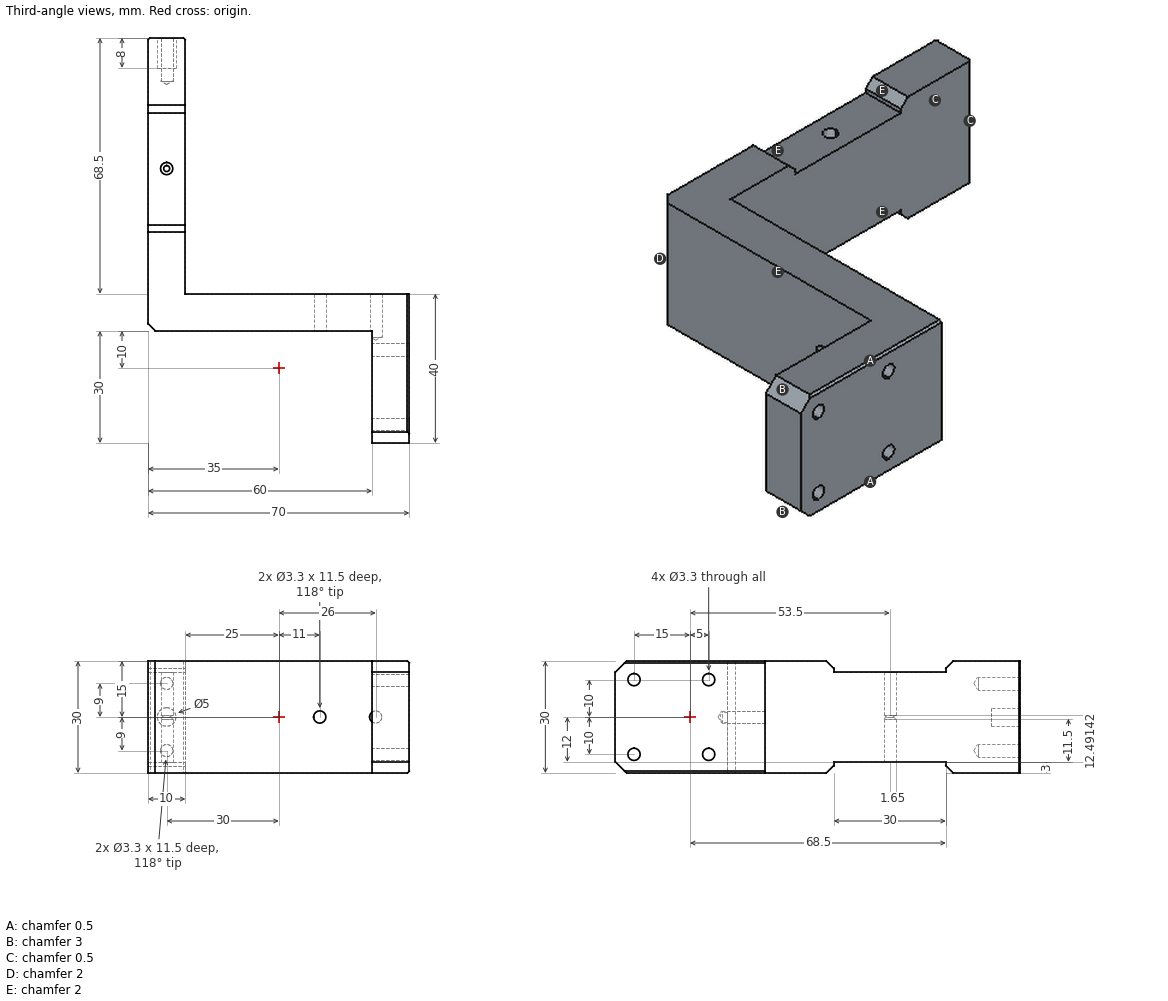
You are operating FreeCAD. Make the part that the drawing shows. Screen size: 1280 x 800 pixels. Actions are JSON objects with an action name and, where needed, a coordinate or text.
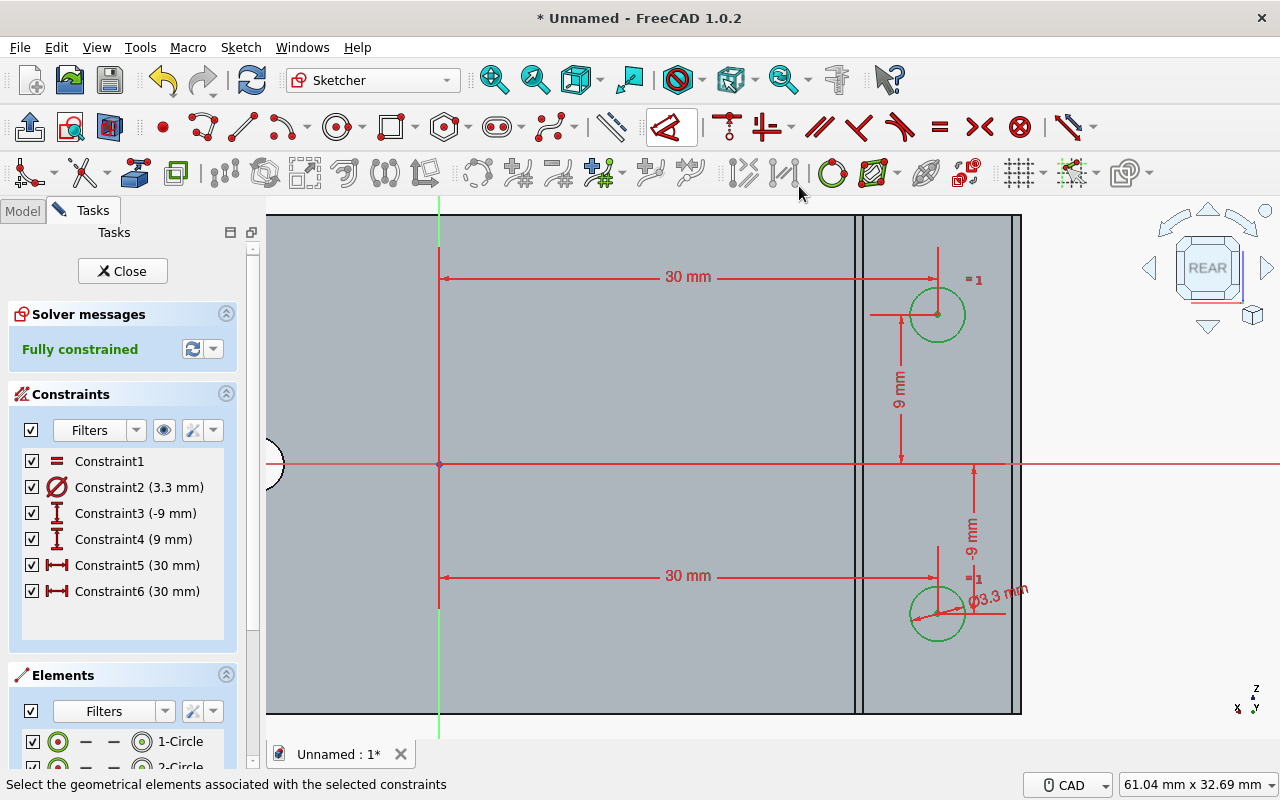
{"action": "left_click", "coordinate": [123, 271]}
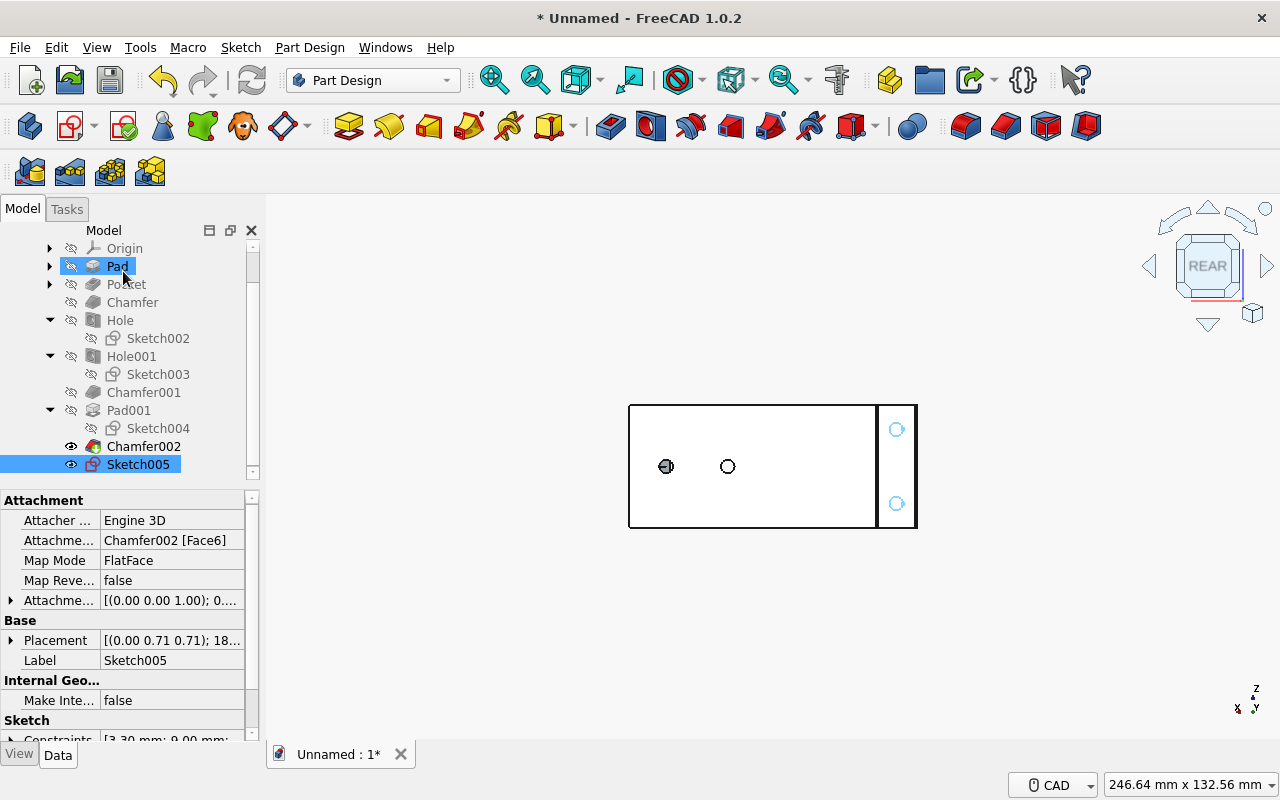
{"action": "left_click", "coordinate": [652, 126]}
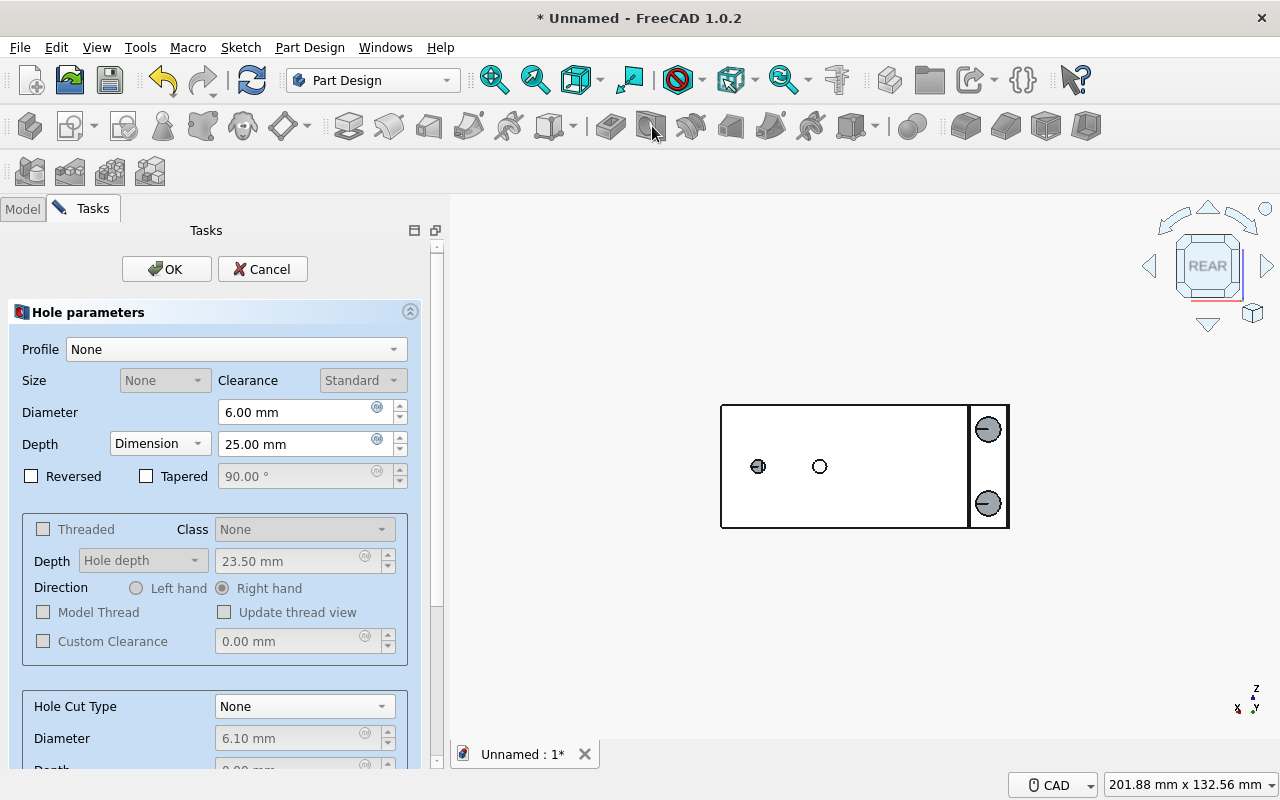
{"action": "triple_click", "coordinate": [305, 412]}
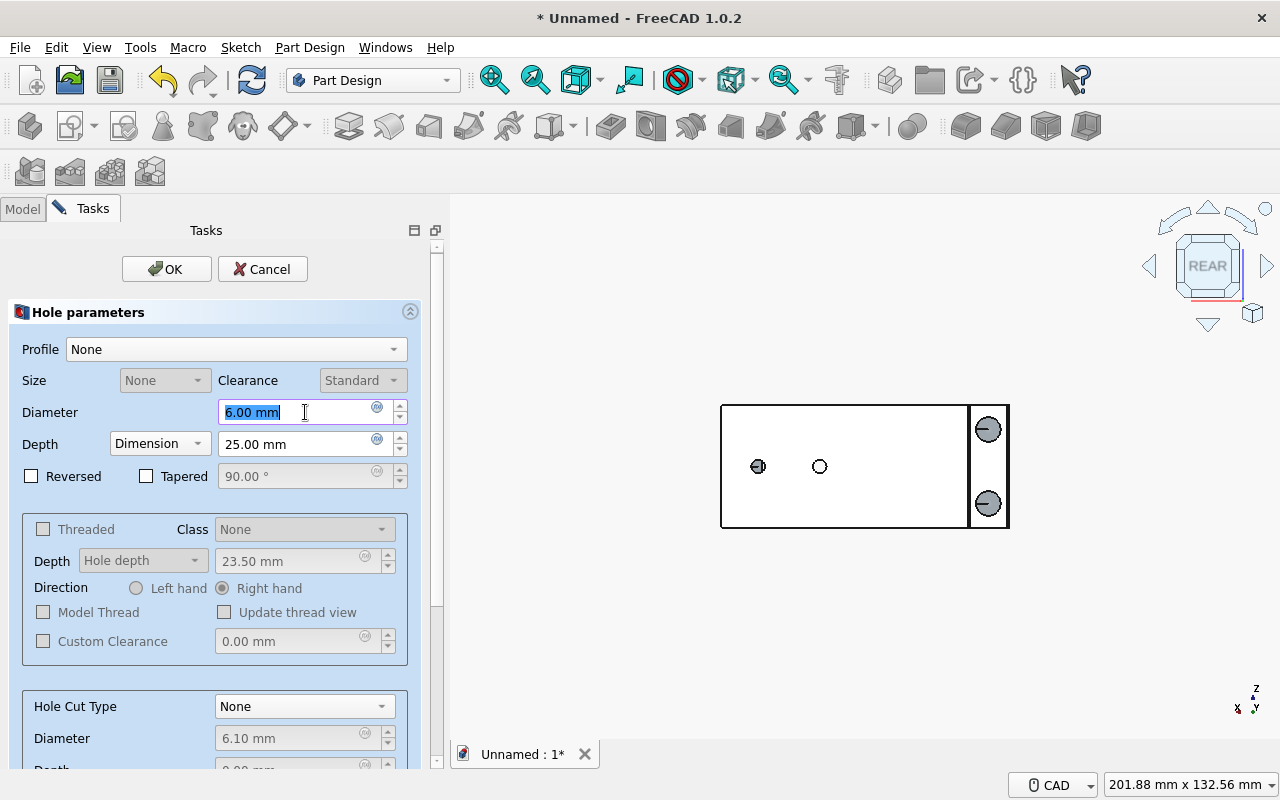
{"action": "type", "text": "3.3"}
{"action": "key", "text": "Tab"}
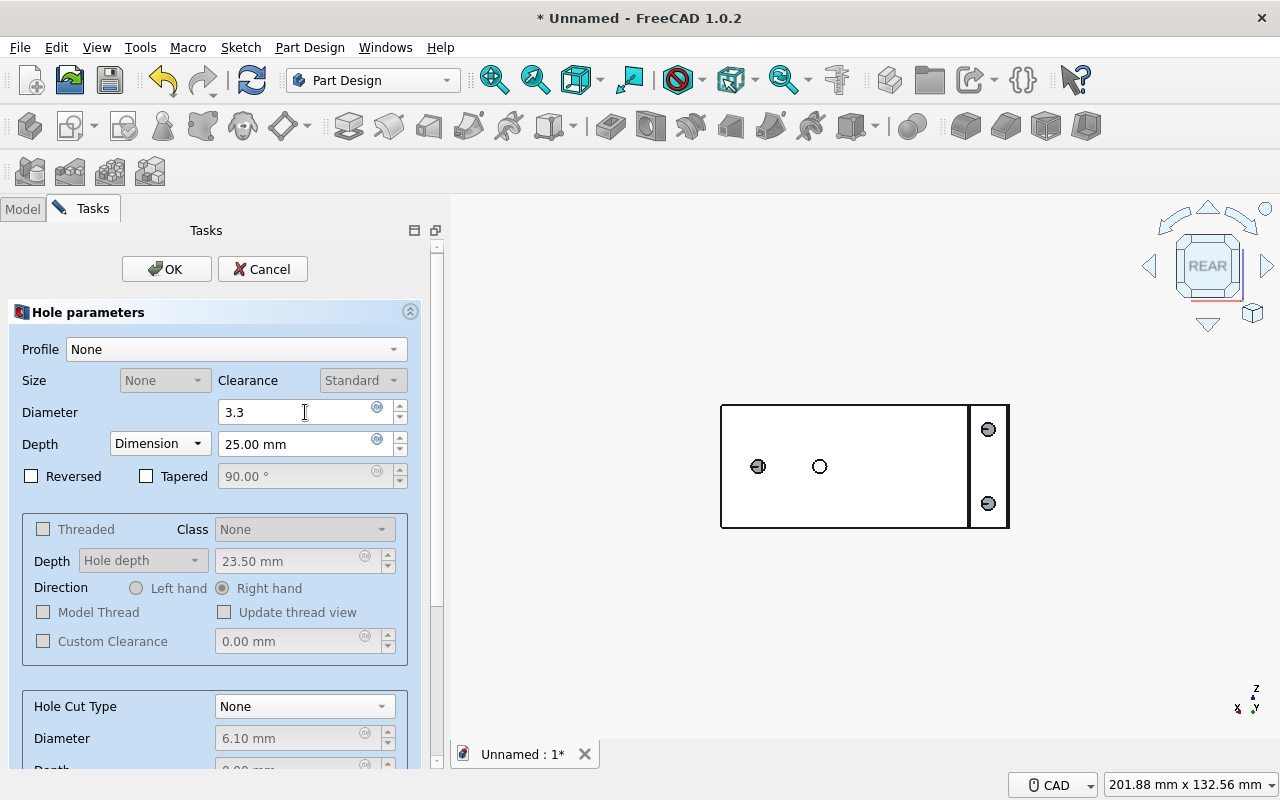
{"action": "triple_click", "coordinate": [305, 444]}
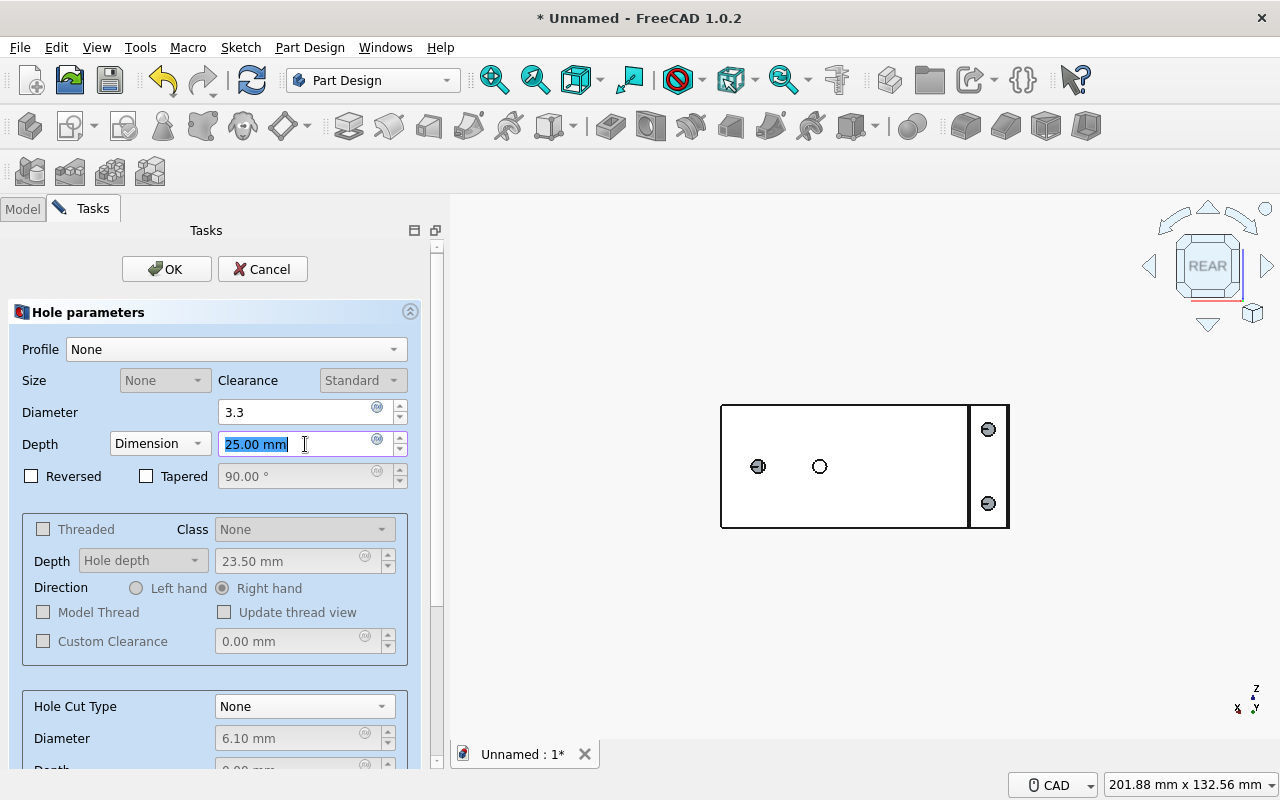
{"action": "type", "text": "11.5"}
{"action": "key", "text": "Tab"}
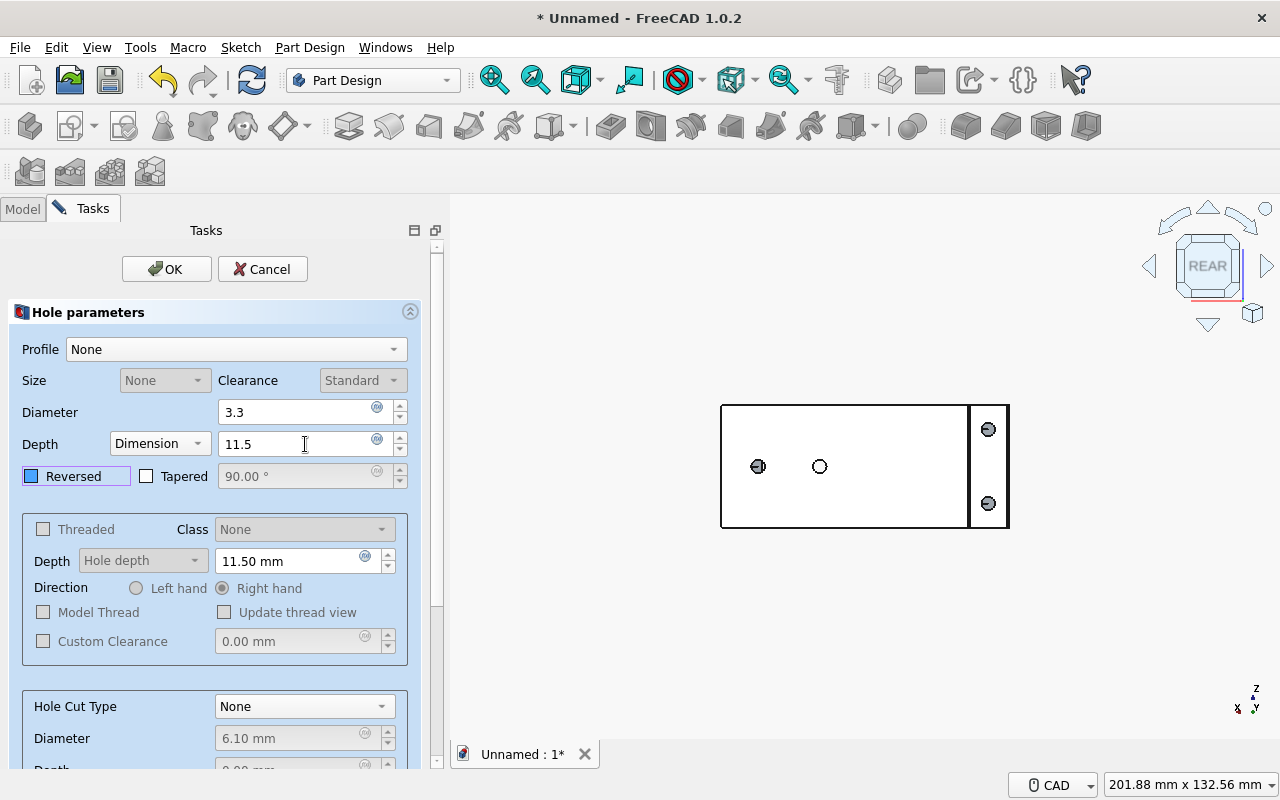
{"action": "left_click", "coordinate": [167, 269]}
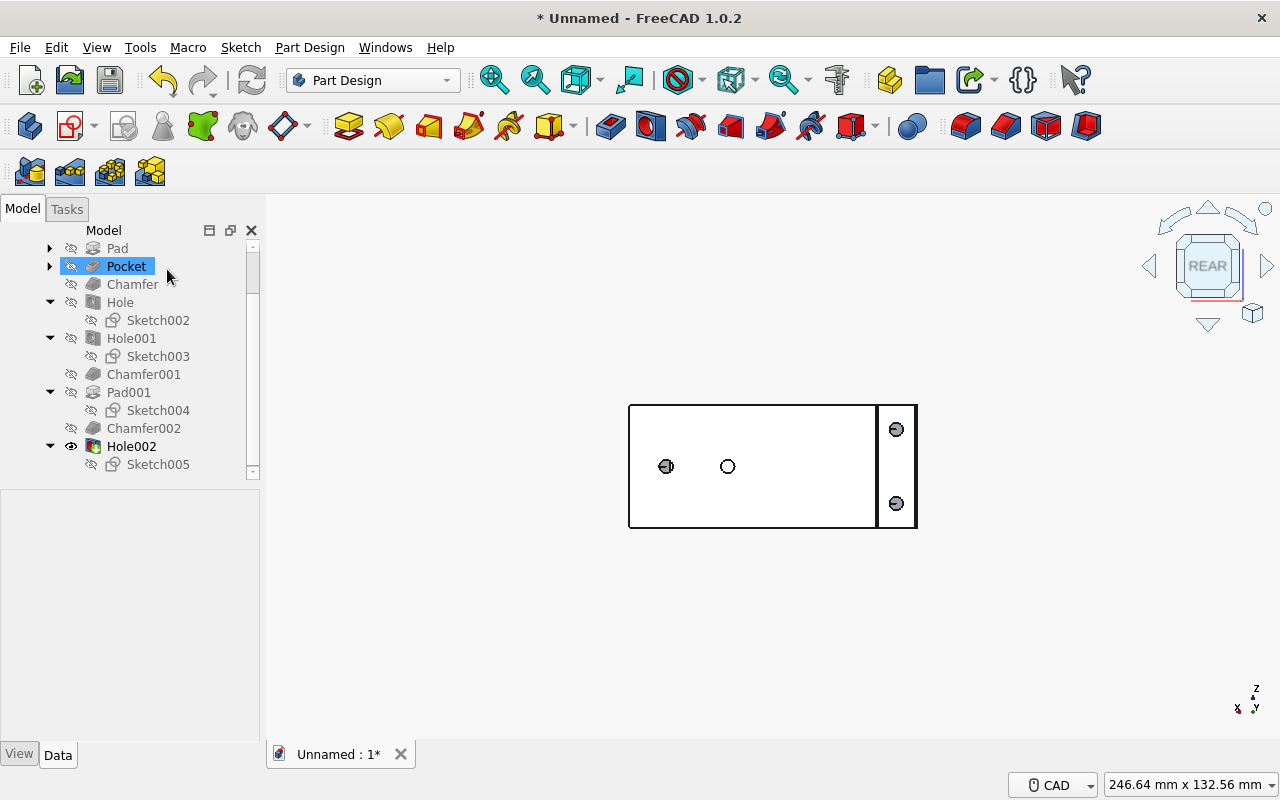
{"action": "left_click", "coordinate": [496, 80]}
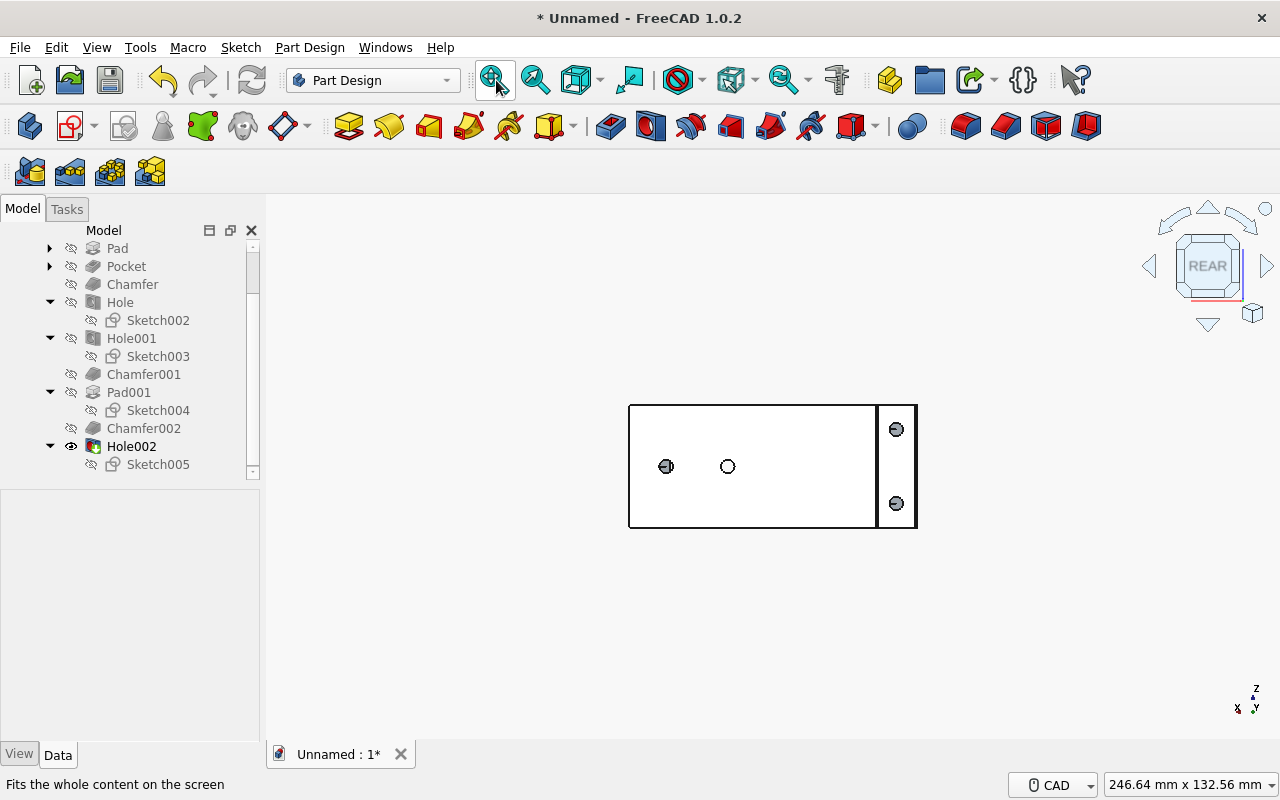
{"action": "key", "text": "0"}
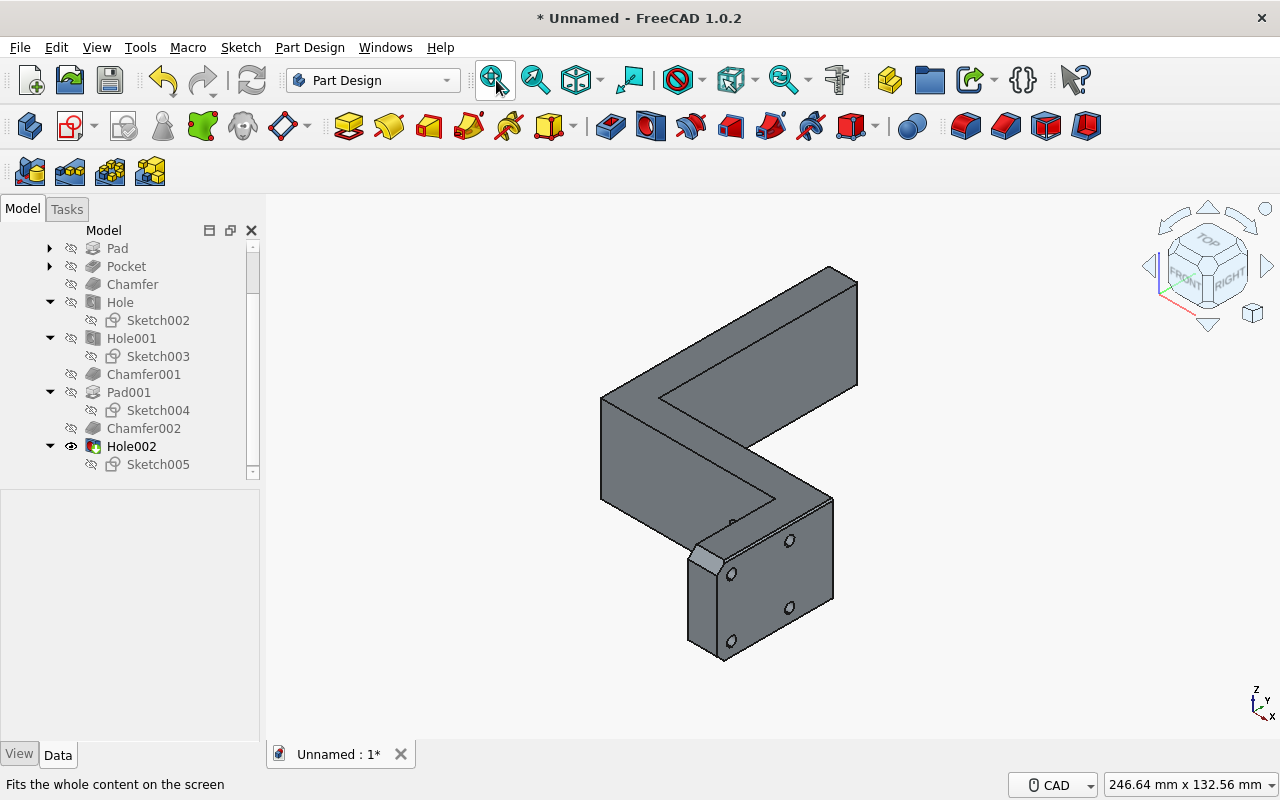
{"action": "key", "text": "2"}